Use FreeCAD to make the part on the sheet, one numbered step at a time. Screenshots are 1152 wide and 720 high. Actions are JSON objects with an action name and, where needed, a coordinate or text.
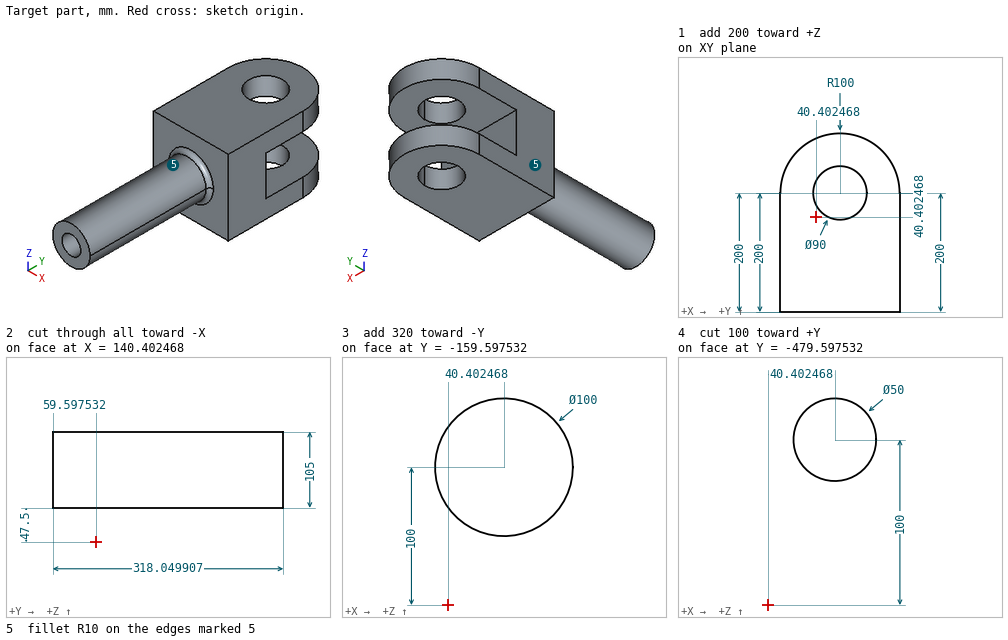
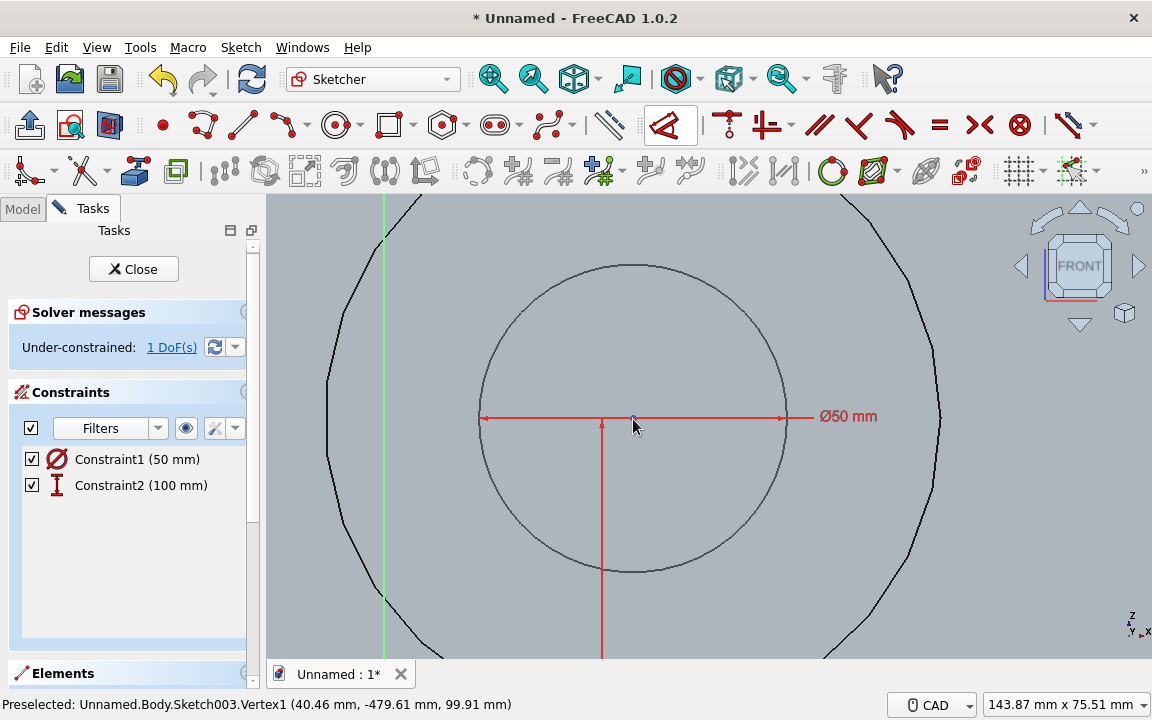
{"action": "left_click", "coordinate": [633, 418]}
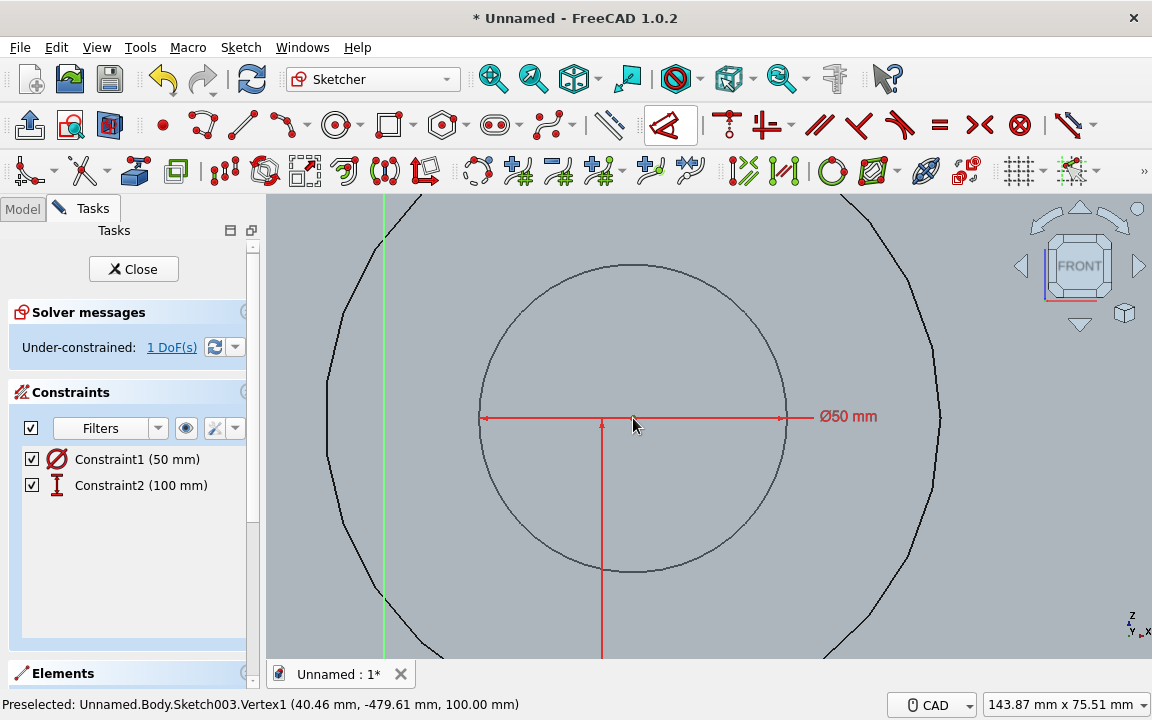
{"action": "key", "text": "l"}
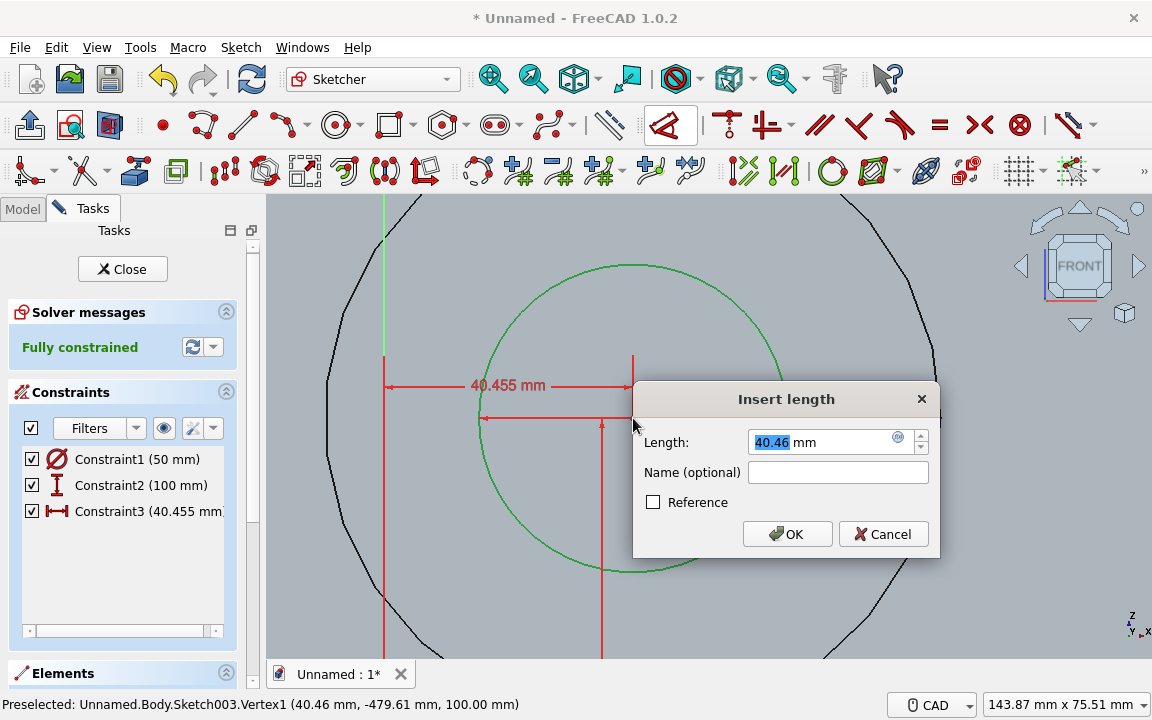
{"action": "type", "text": "40.402468"}
{"action": "key", "text": "Return"}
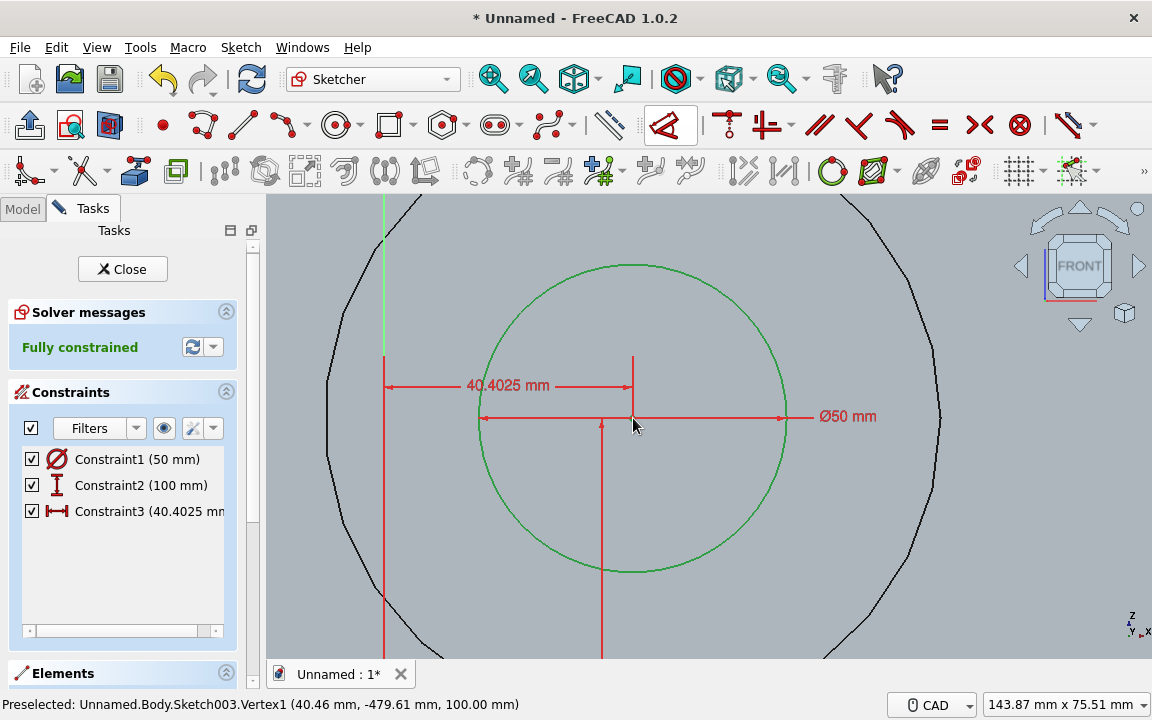
{"action": "left_click", "coordinate": [123, 269]}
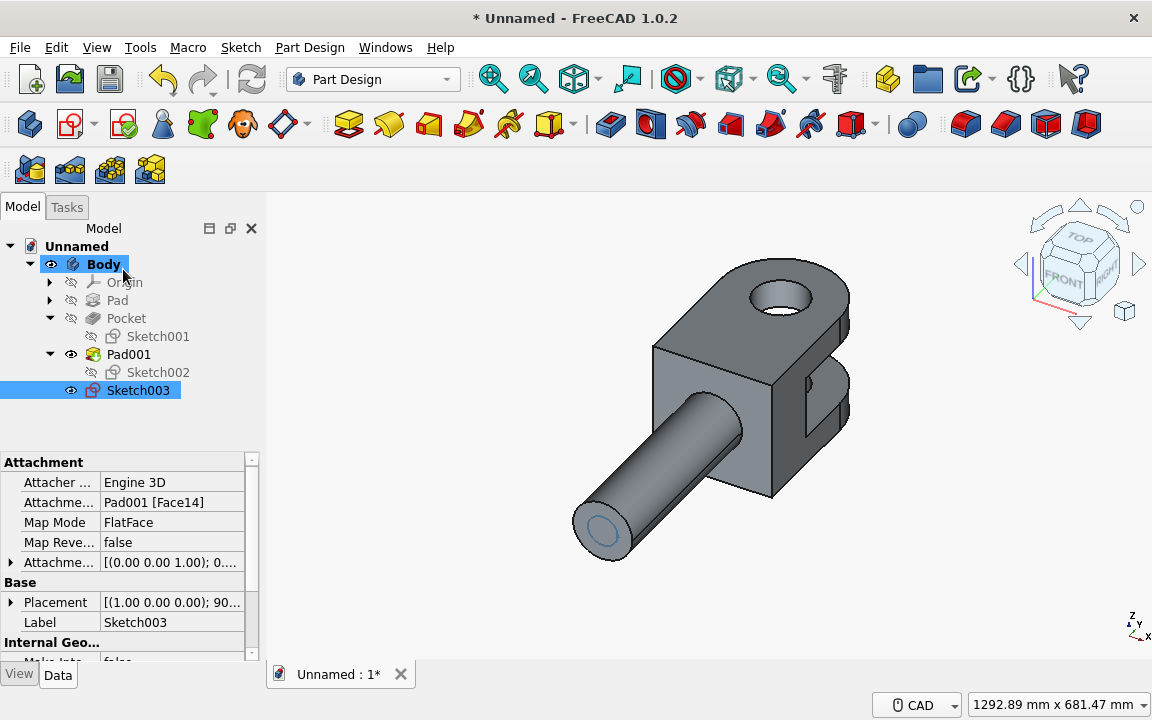
{"action": "left_click", "coordinate": [612, 124]}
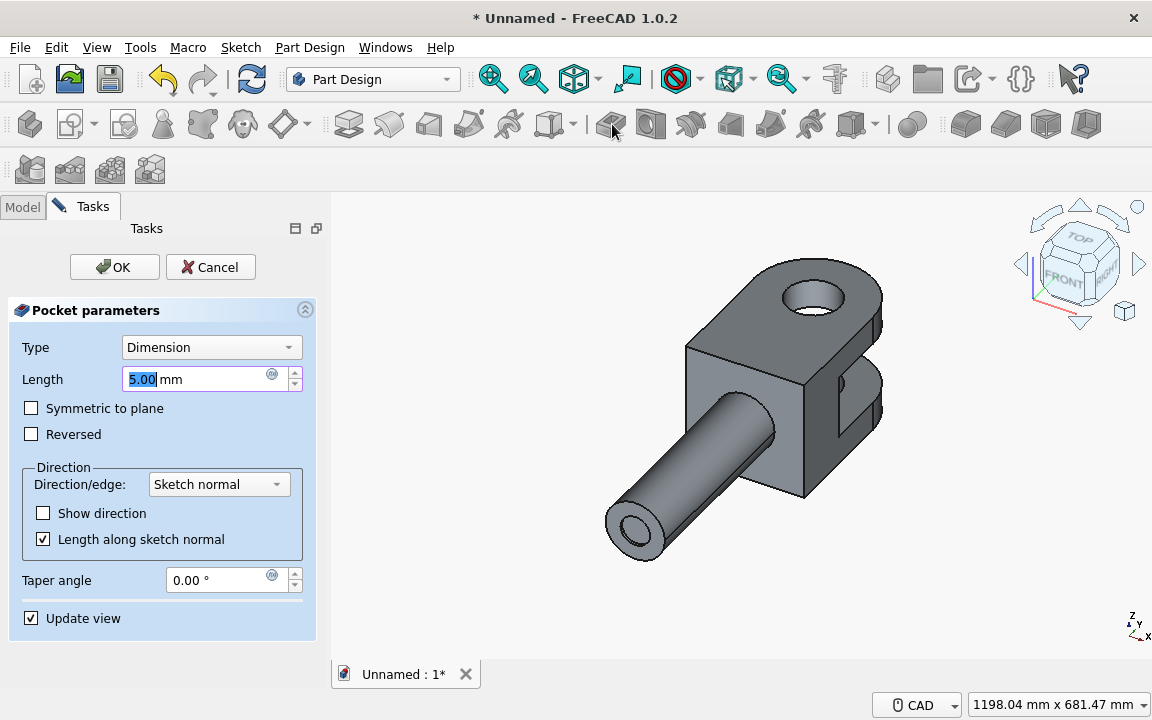
{"action": "type", "text": "100"}
{"action": "key", "text": "Tab"}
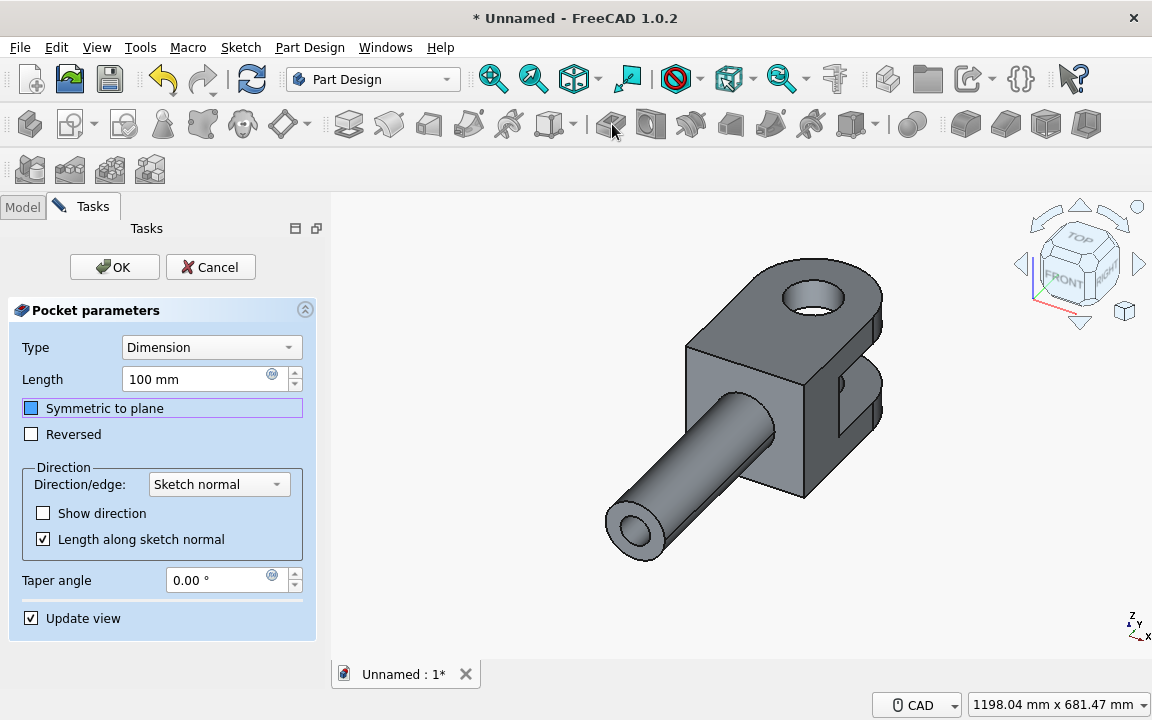
{"action": "left_click", "coordinate": [115, 267]}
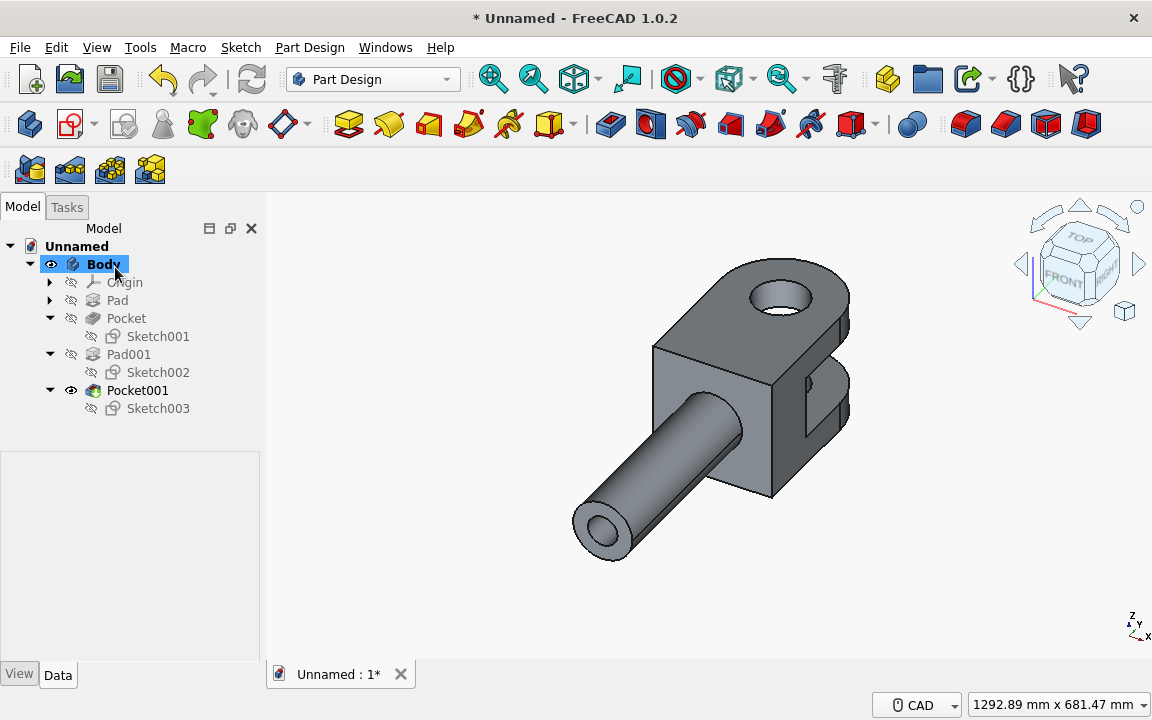
{"action": "key", "text": "0"}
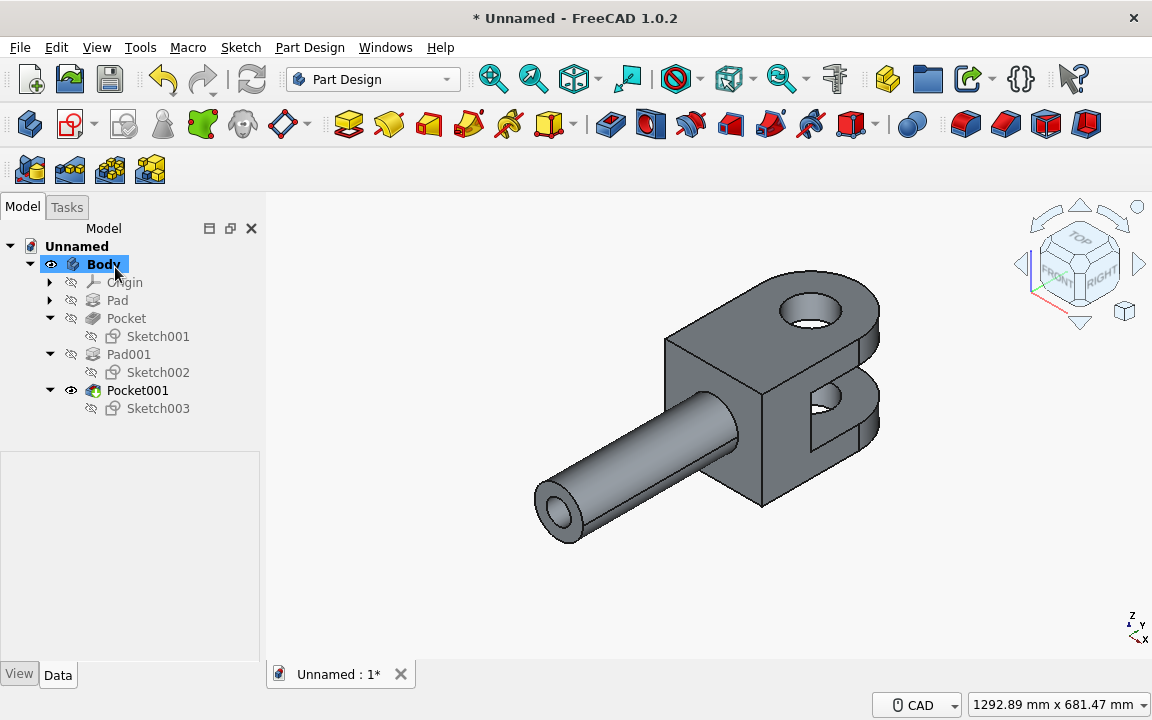
{"action": "key", "text": "2"}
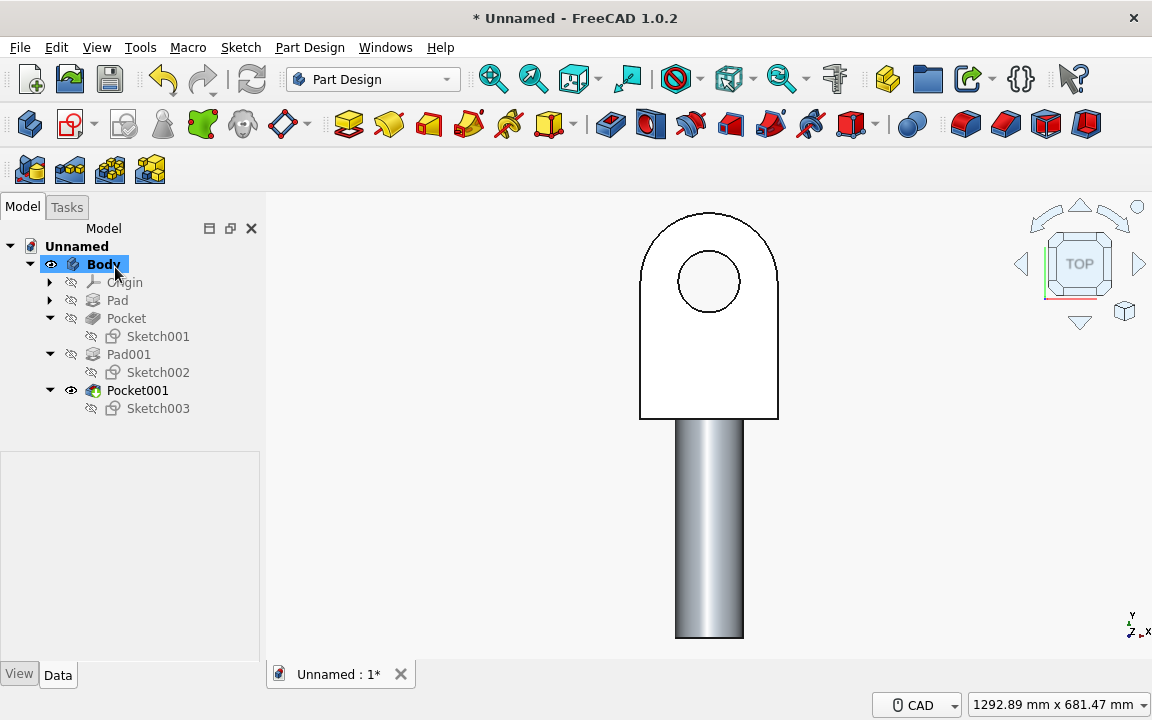
{"action": "key", "text": "1"}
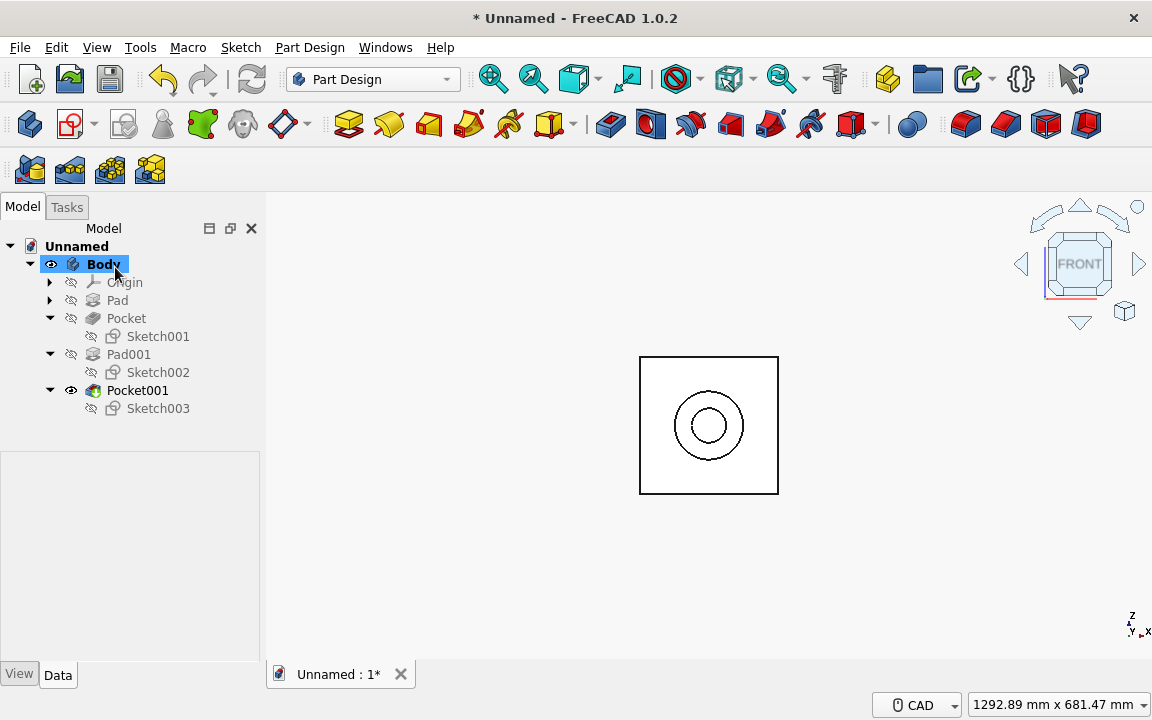
{"action": "key", "text": "v f"}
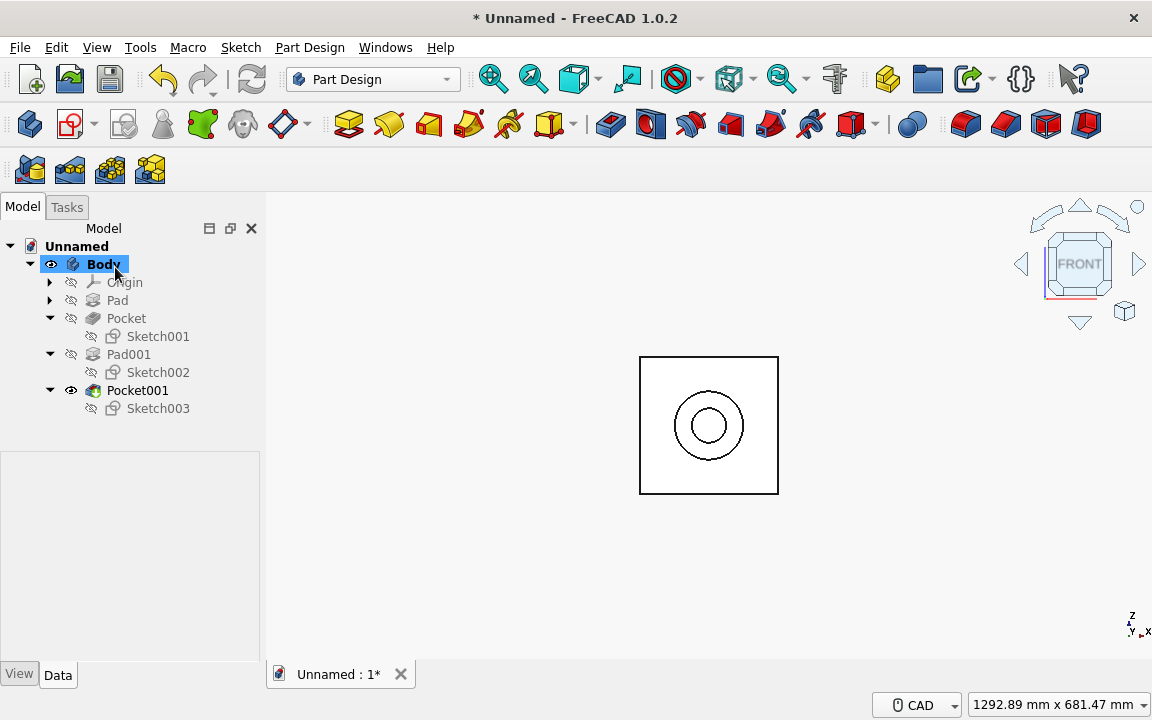
{"action": "key", "text": "3"}